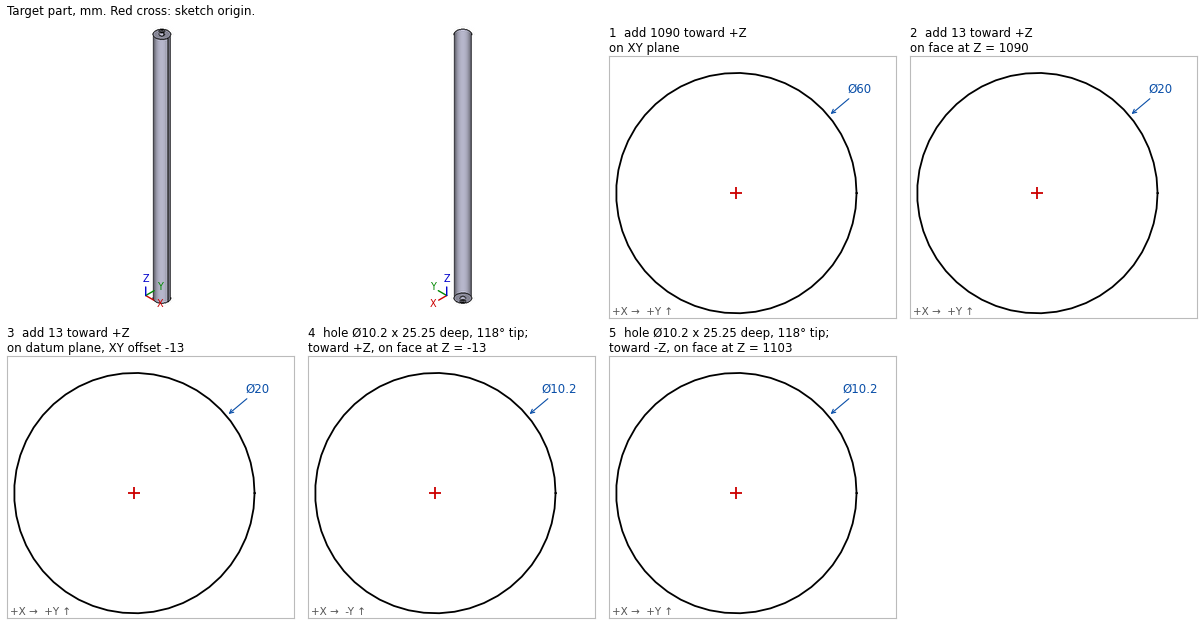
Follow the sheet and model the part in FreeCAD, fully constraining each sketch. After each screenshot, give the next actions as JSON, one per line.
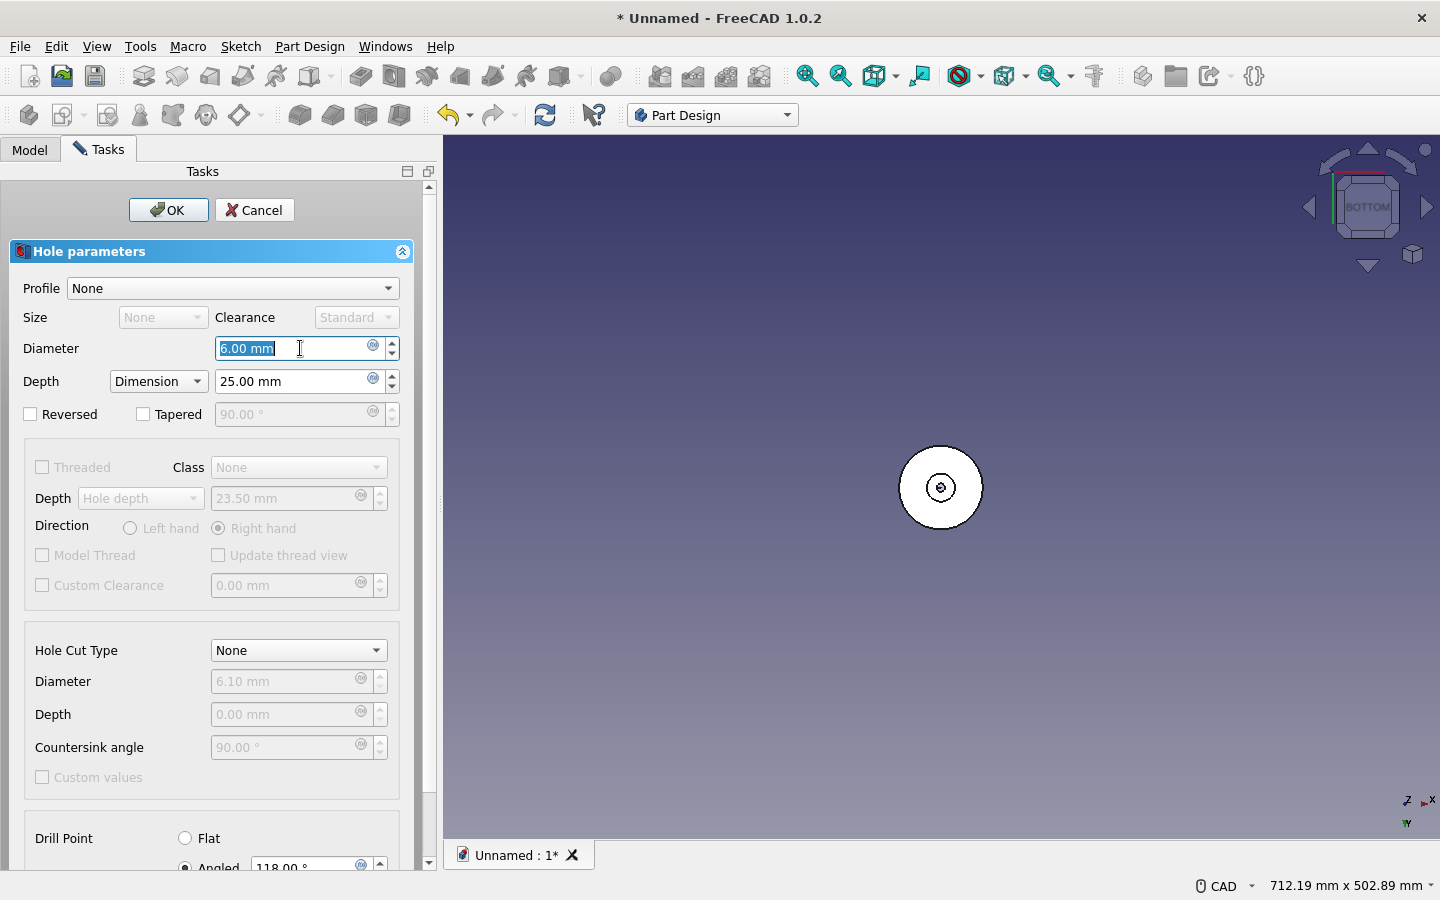
{"action": "type", "text": "10.2"}
{"action": "key", "text": "Tab"}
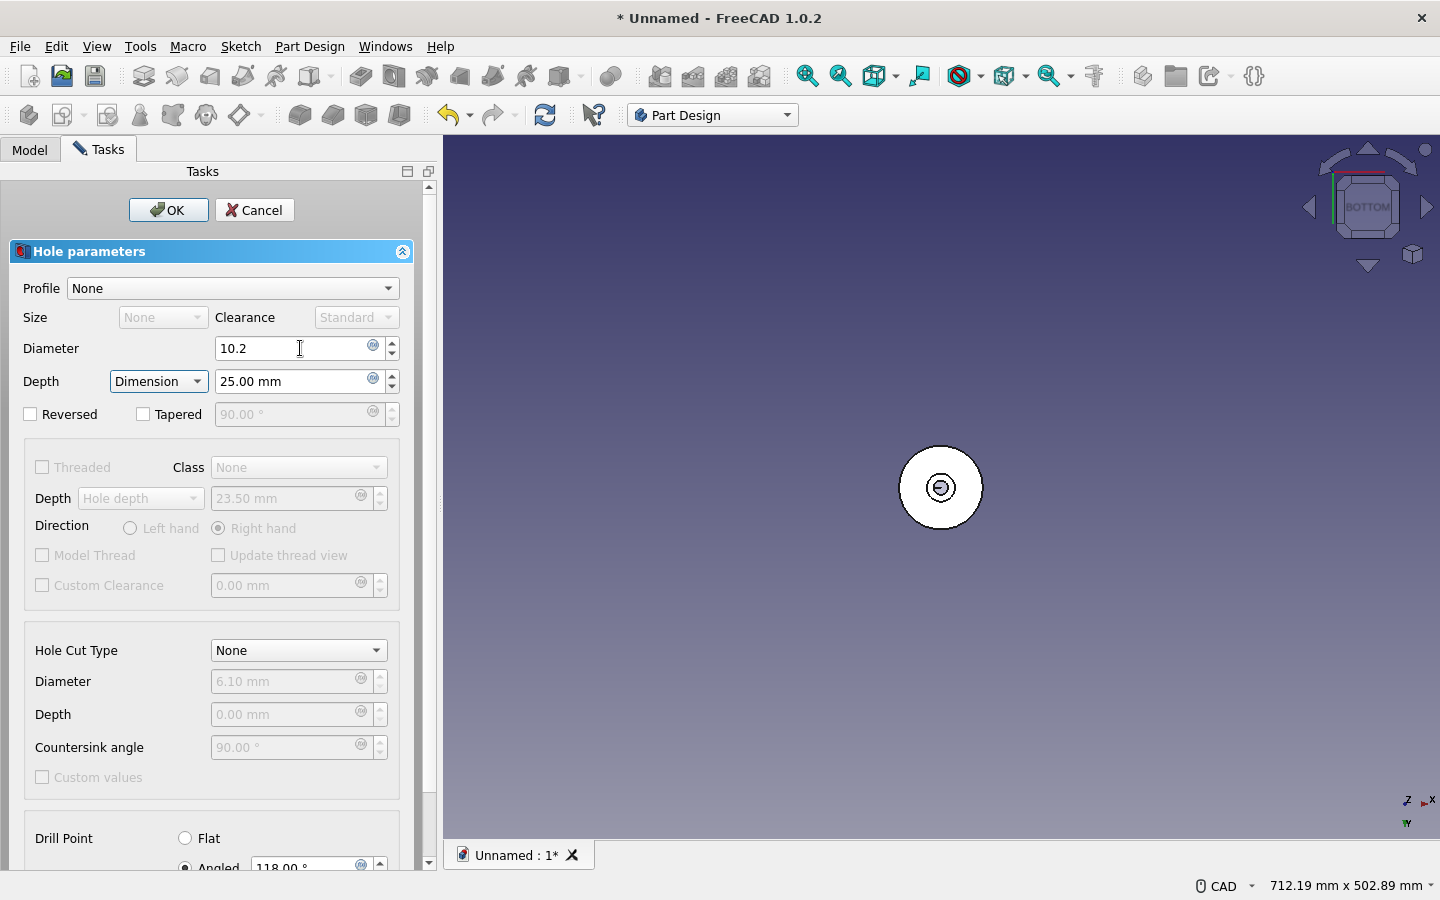
{"action": "triple_click", "coordinate": [300, 382]}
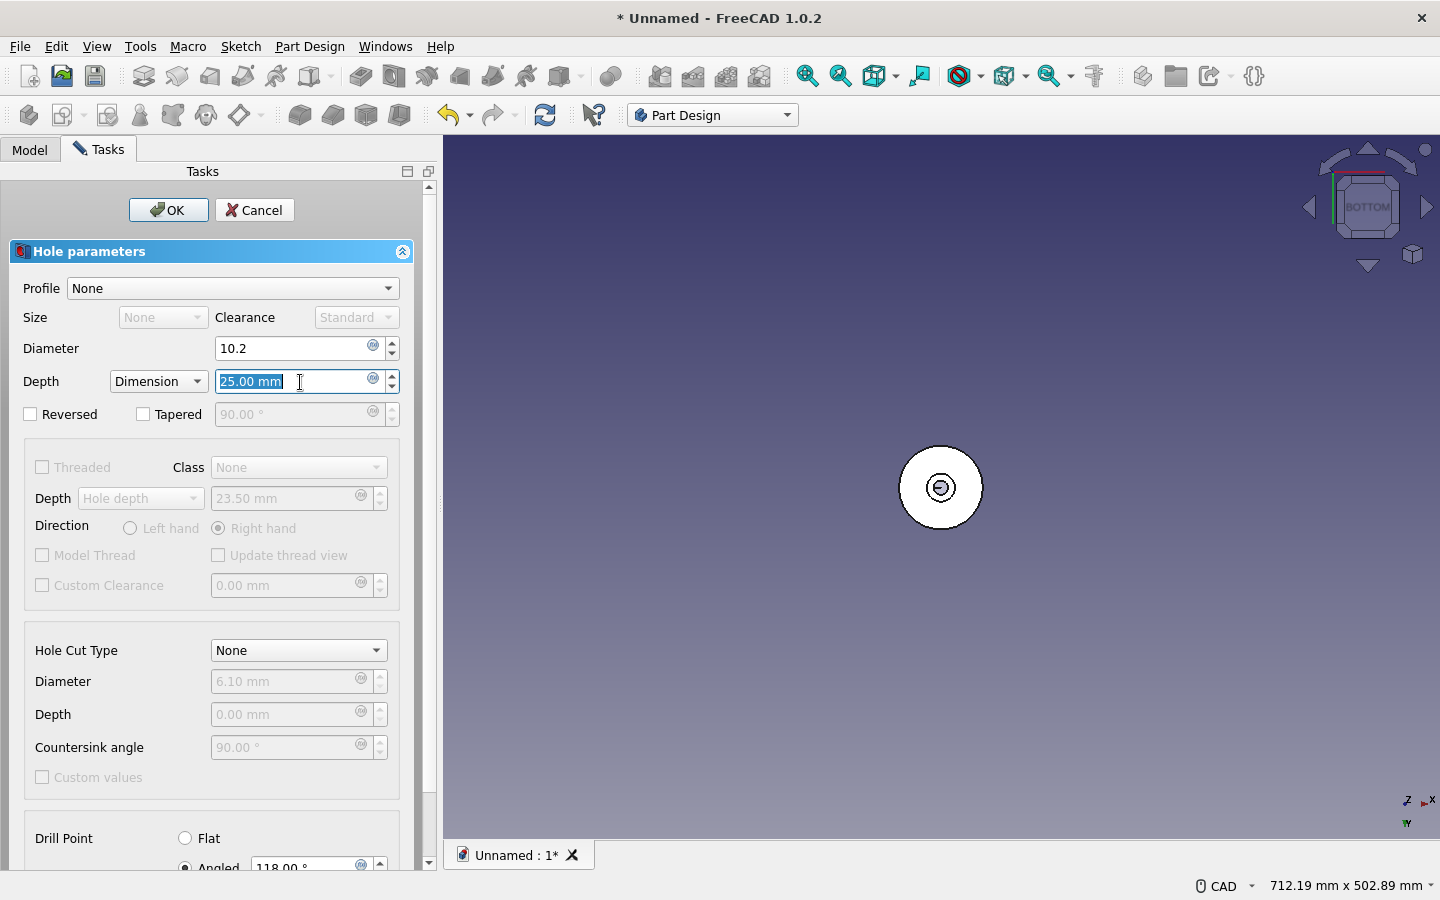
{"action": "type", "text": "25.25"}
{"action": "key", "text": "Tab"}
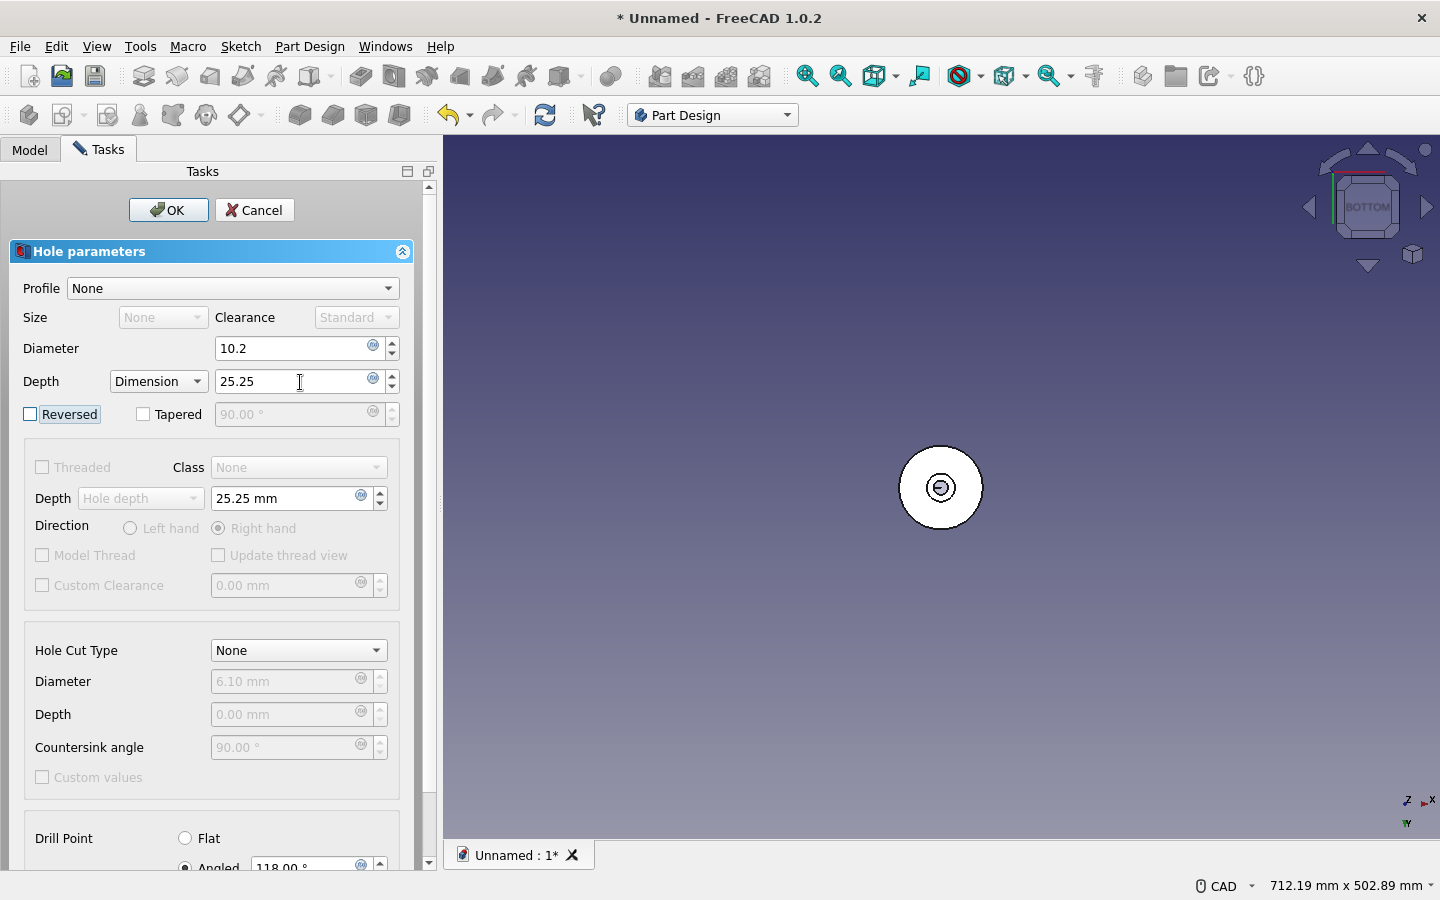
{"action": "left_click", "coordinate": [169, 210]}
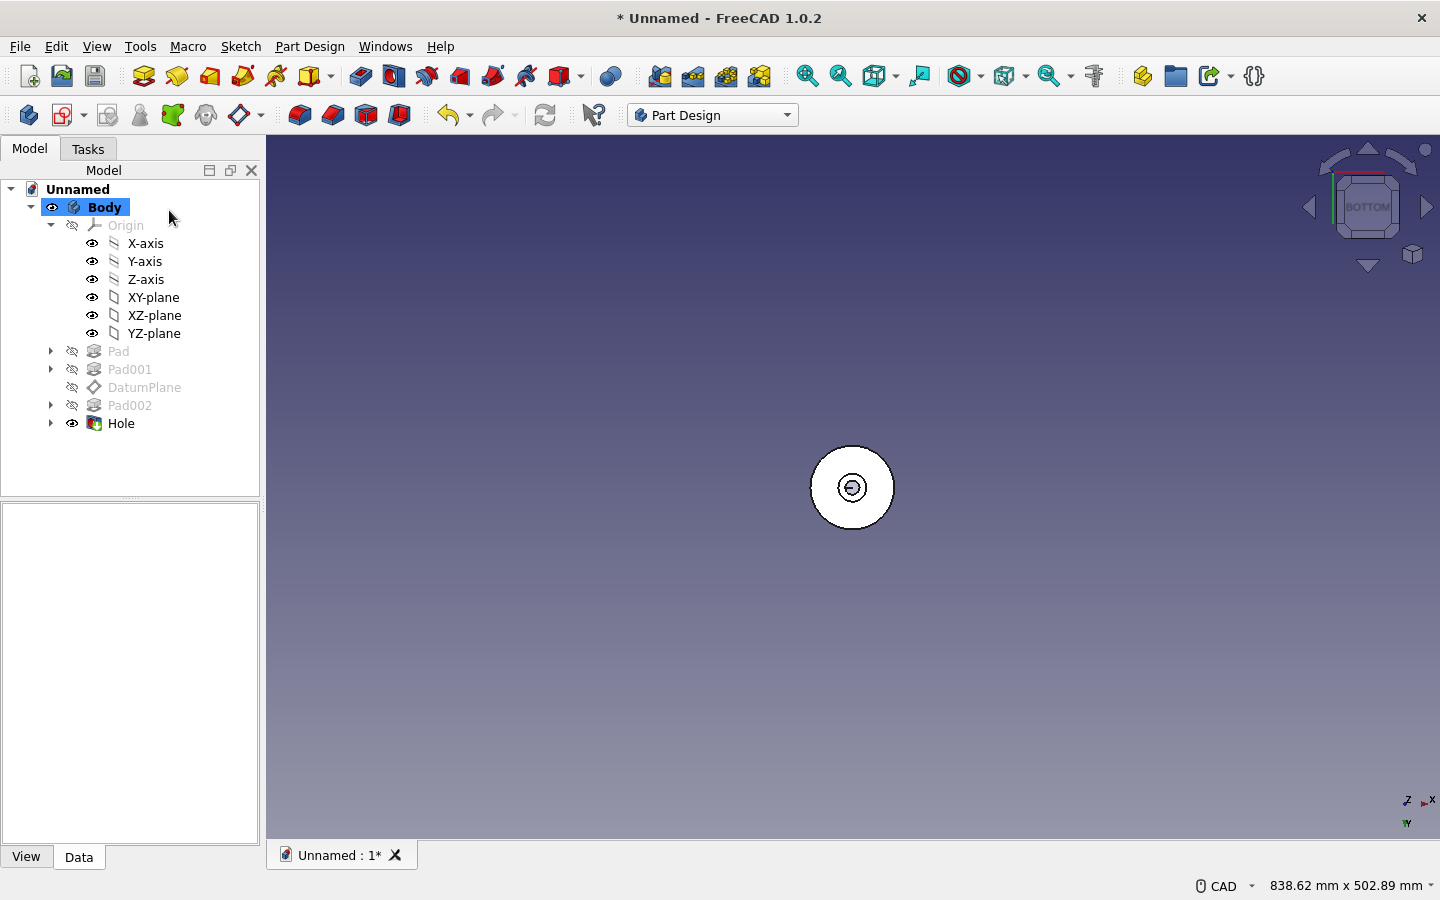
{"action": "key", "text": "v f"}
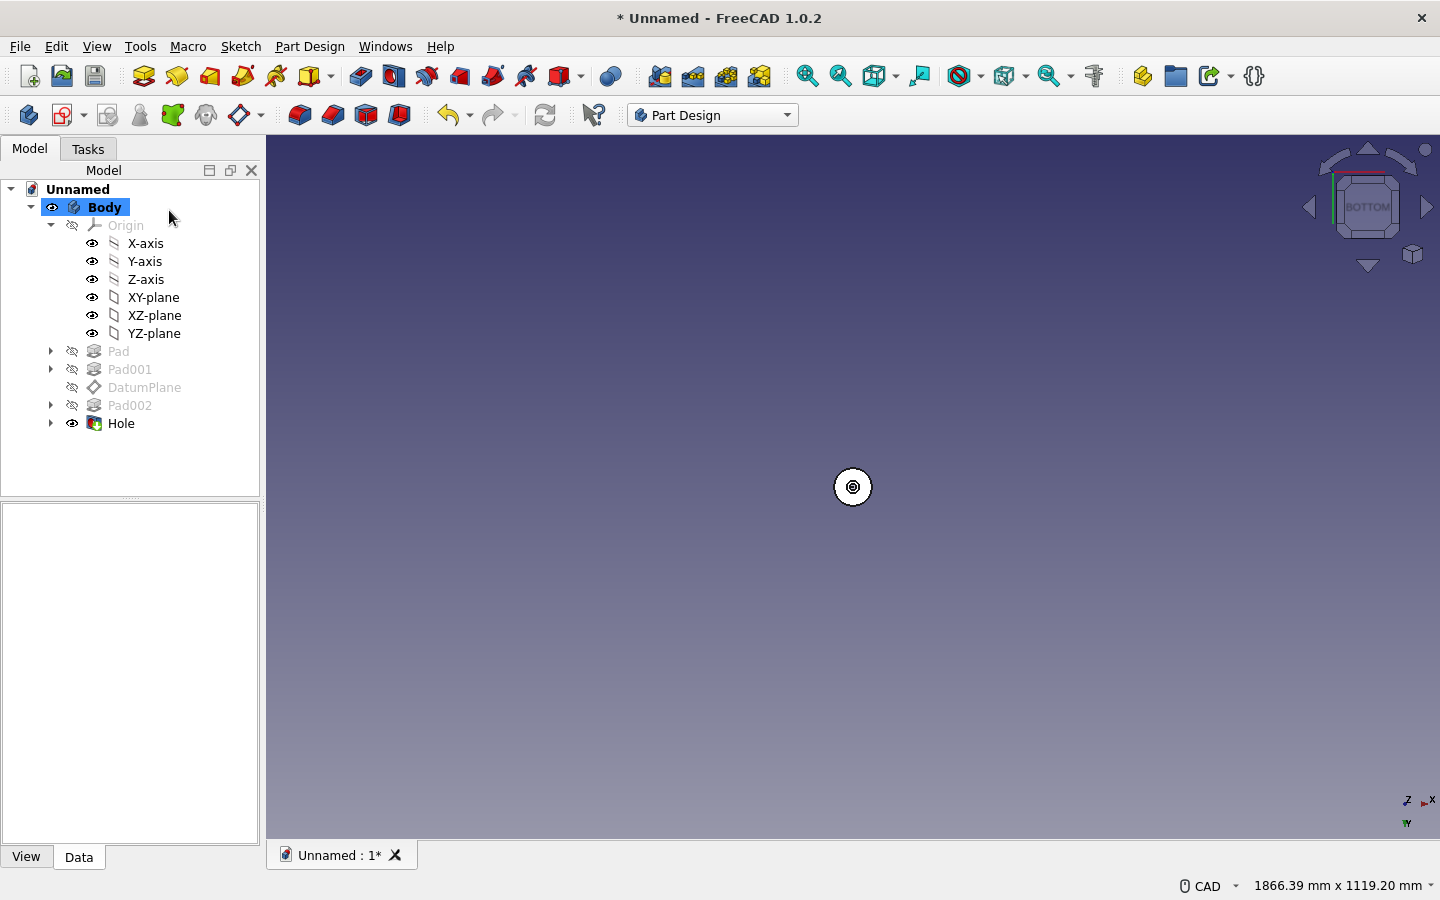
{"action": "key", "text": "0"}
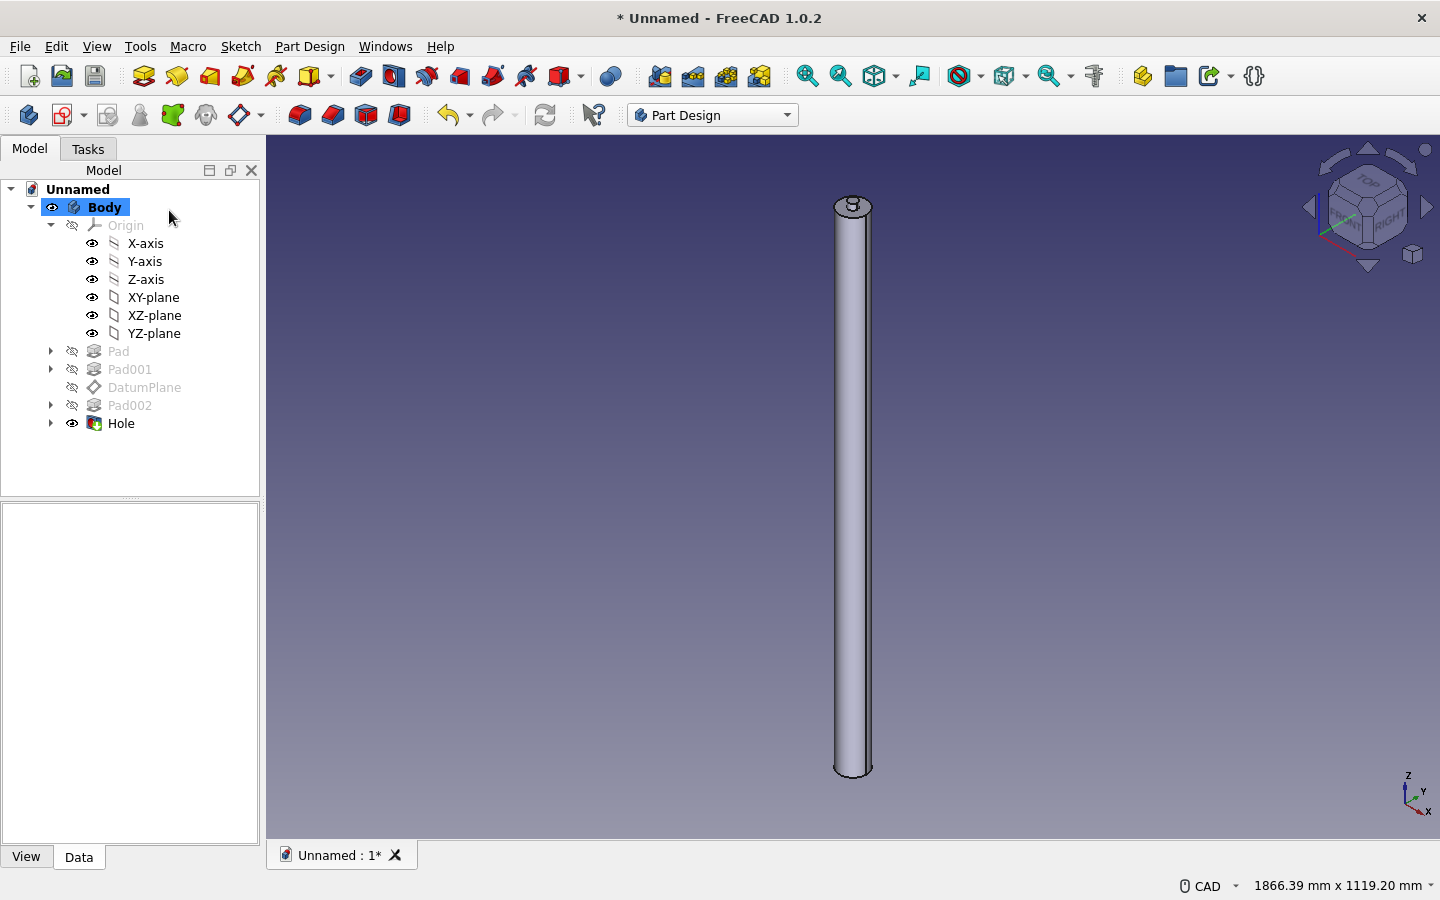
{"action": "scroll", "coordinate": [853, 199], "scroll_direction": "up", "scroll_amount": 4}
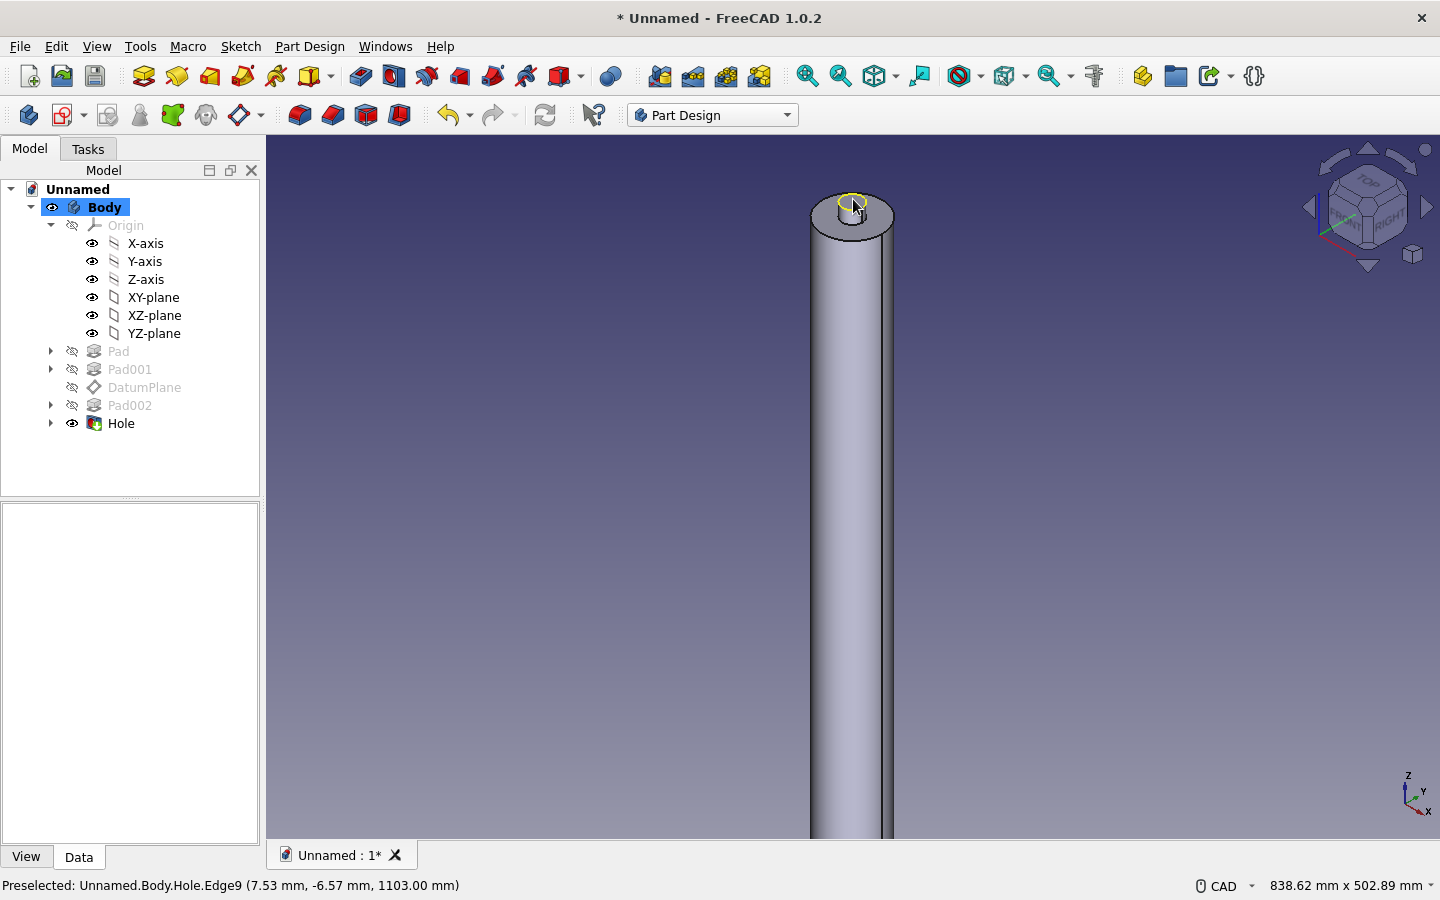
{"action": "left_click", "coordinate": [850, 199]}